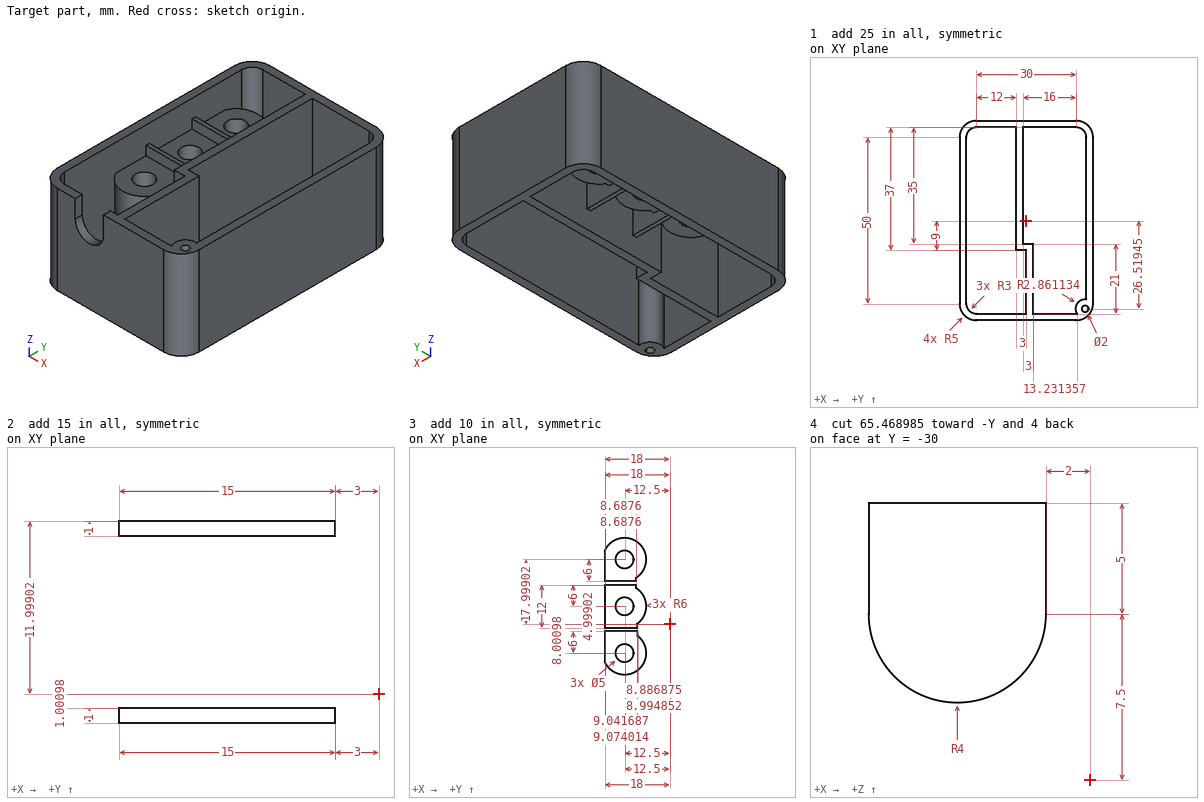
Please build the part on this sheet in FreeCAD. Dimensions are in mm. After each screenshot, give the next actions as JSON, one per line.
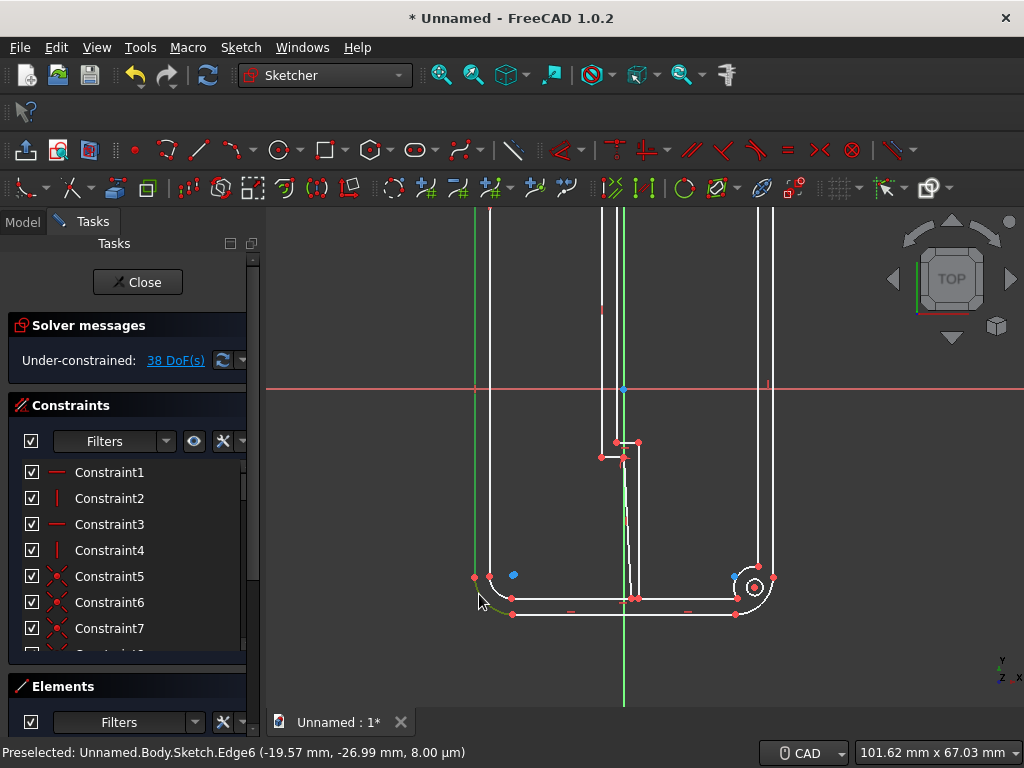
{"action": "left_click", "coordinate": [756, 150]}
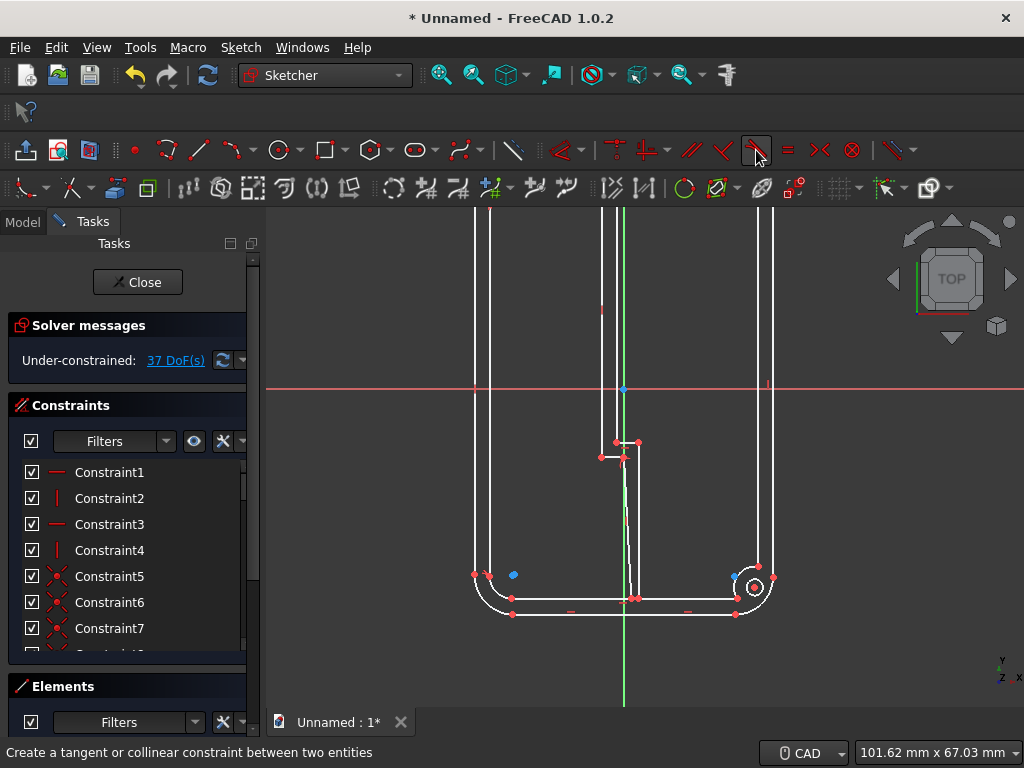
{"action": "left_click", "coordinate": [579, 615]}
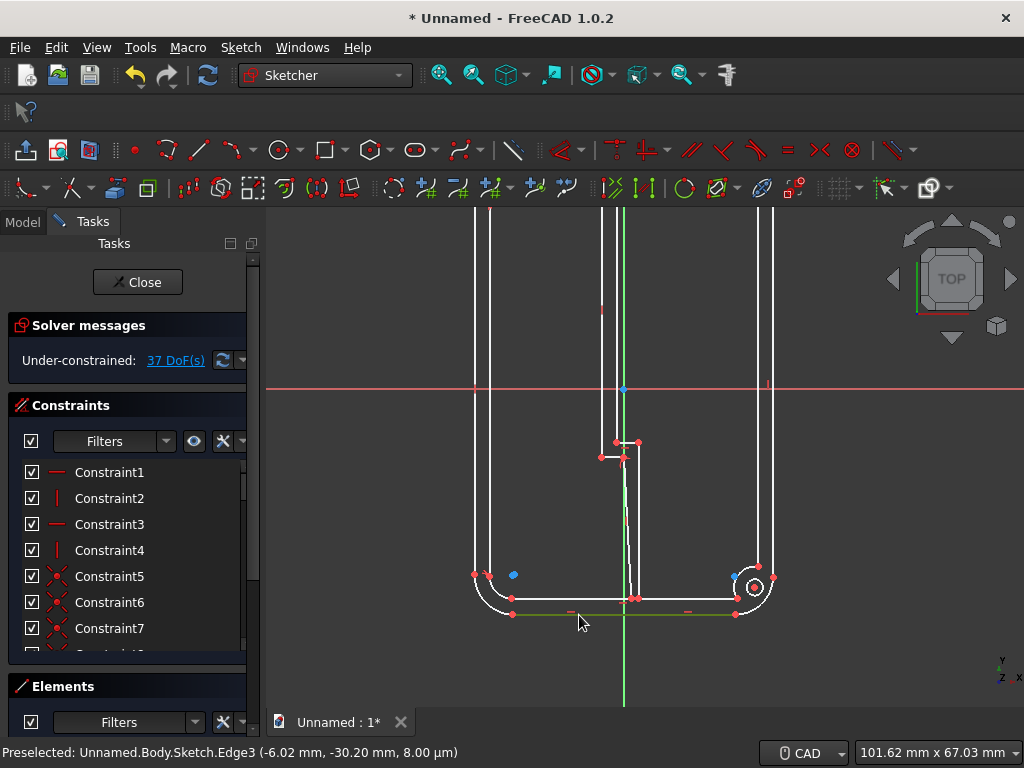
{"action": "left_click", "coordinate": [479, 592]}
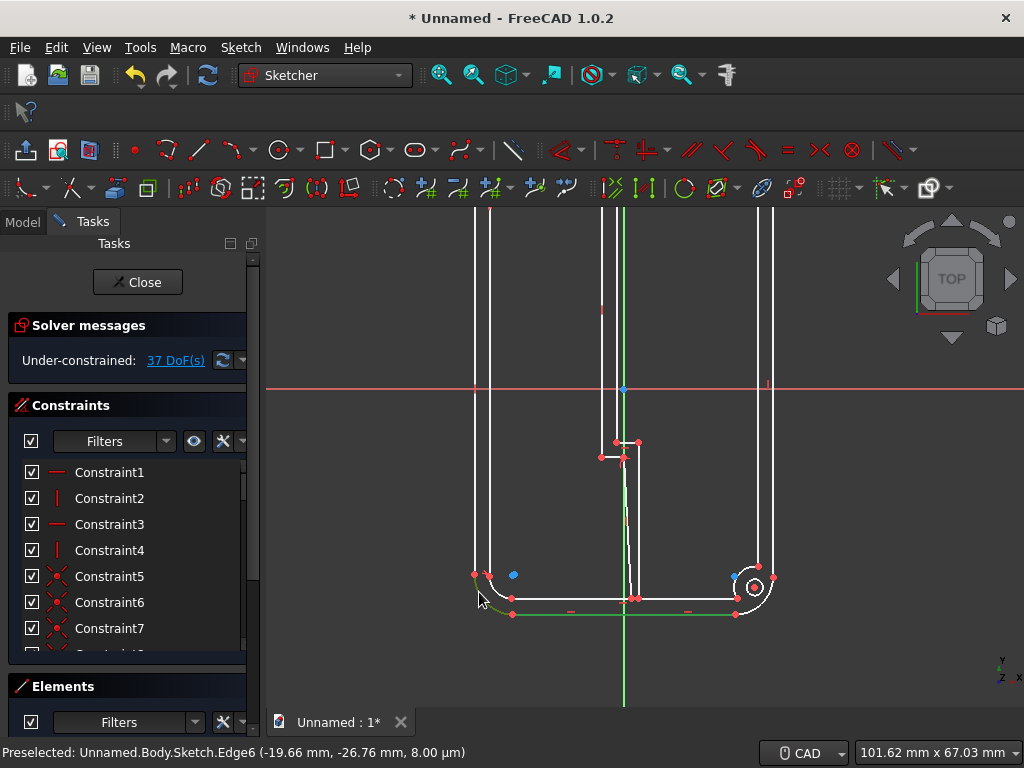
{"action": "left_click", "coordinate": [756, 150]}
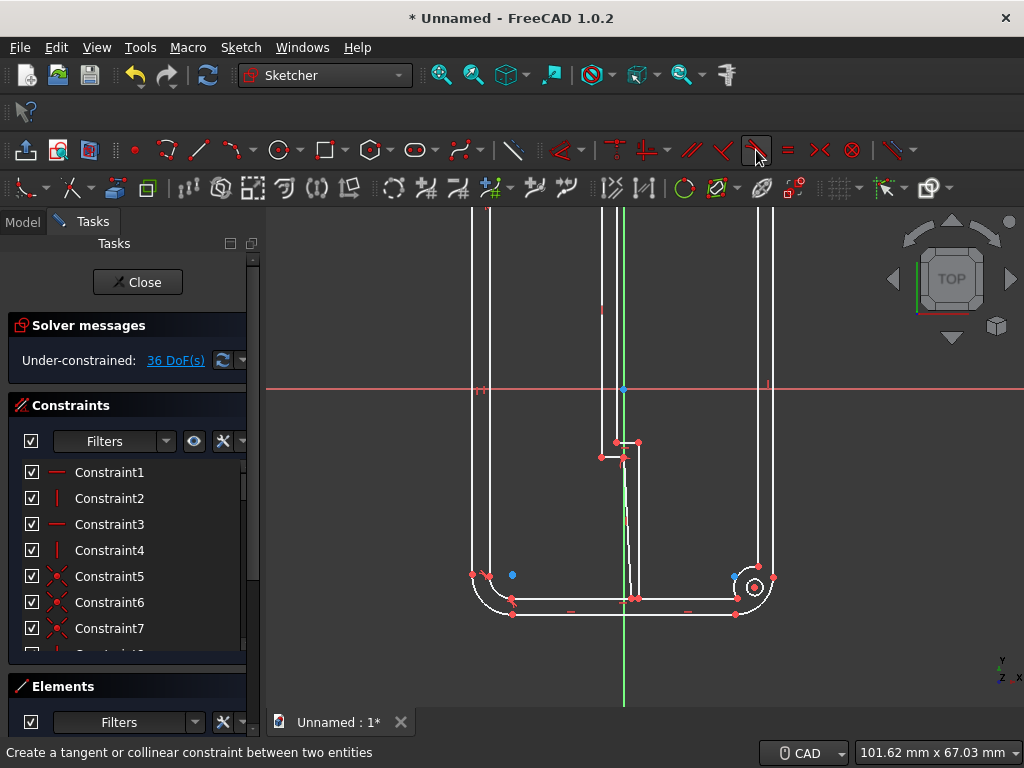
{"action": "left_click", "coordinate": [579, 615]}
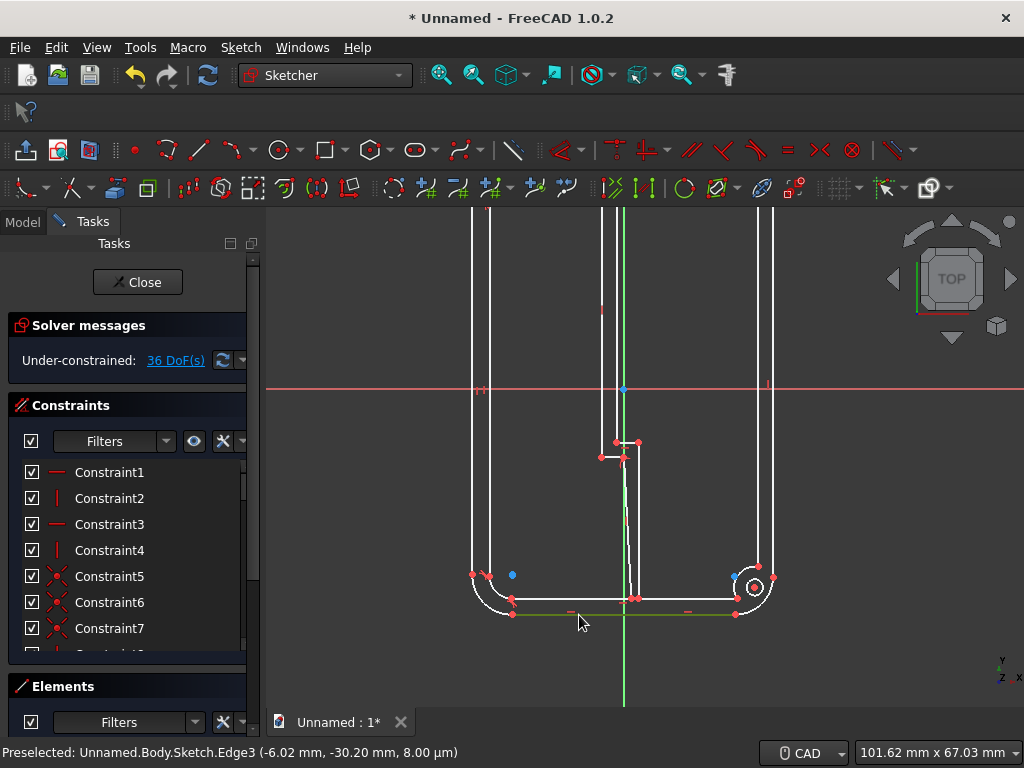
{"action": "left_click", "coordinate": [753, 610]}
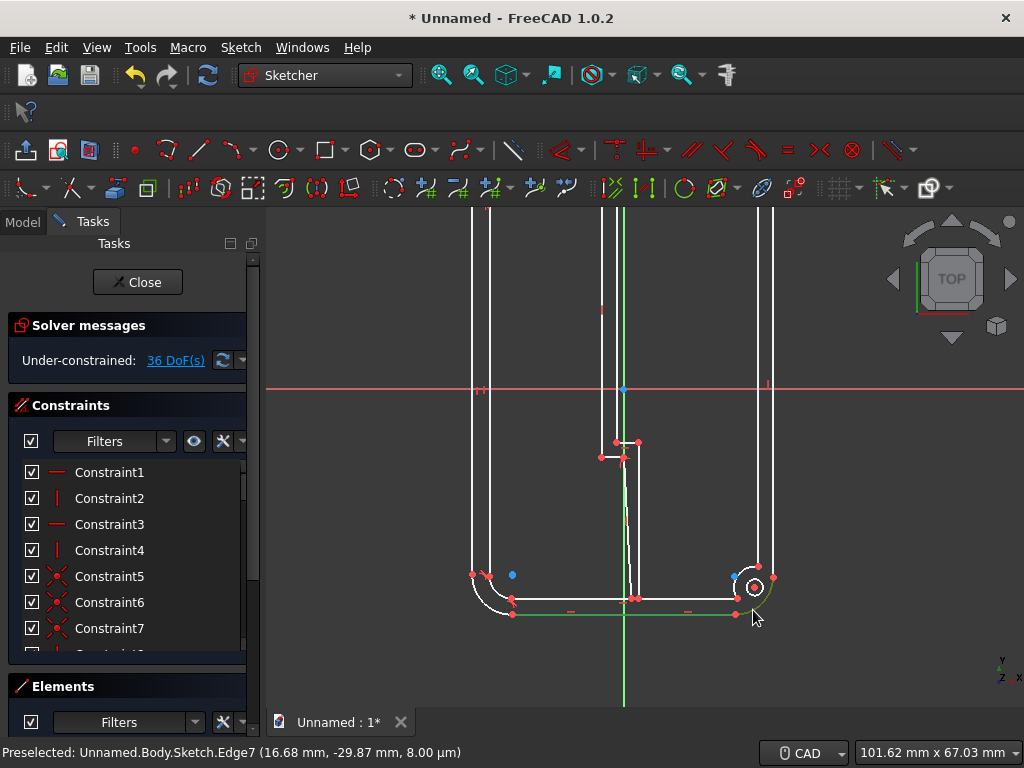
{"action": "left_click", "coordinate": [756, 150]}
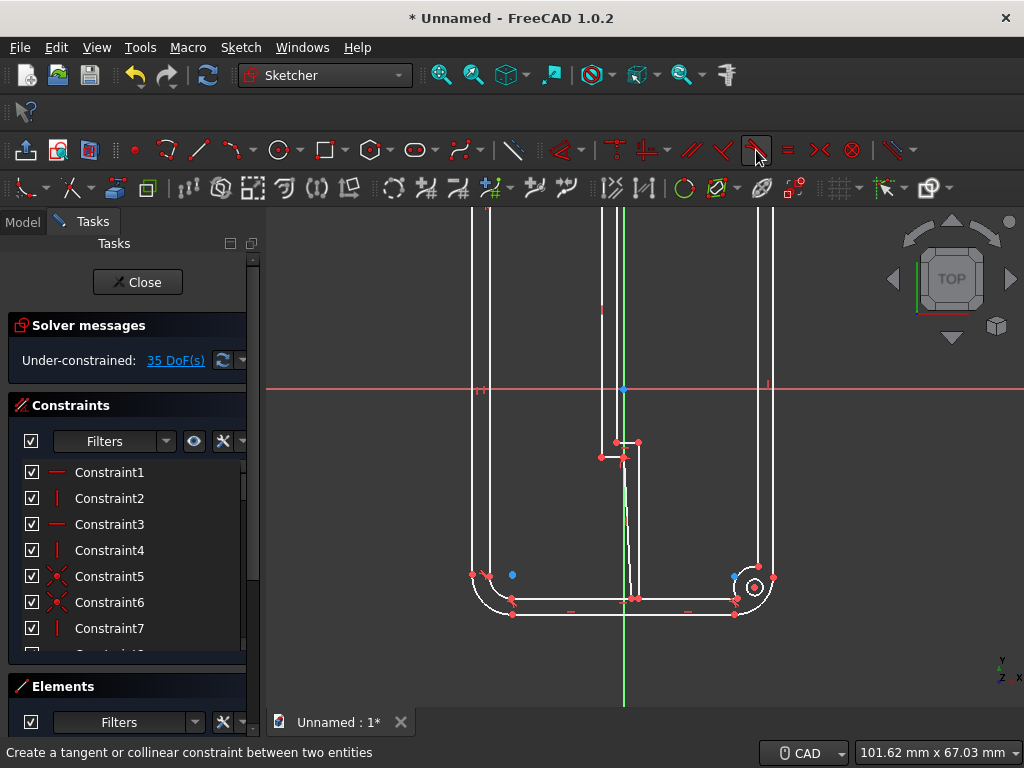
{"action": "left_click", "coordinate": [773, 466]}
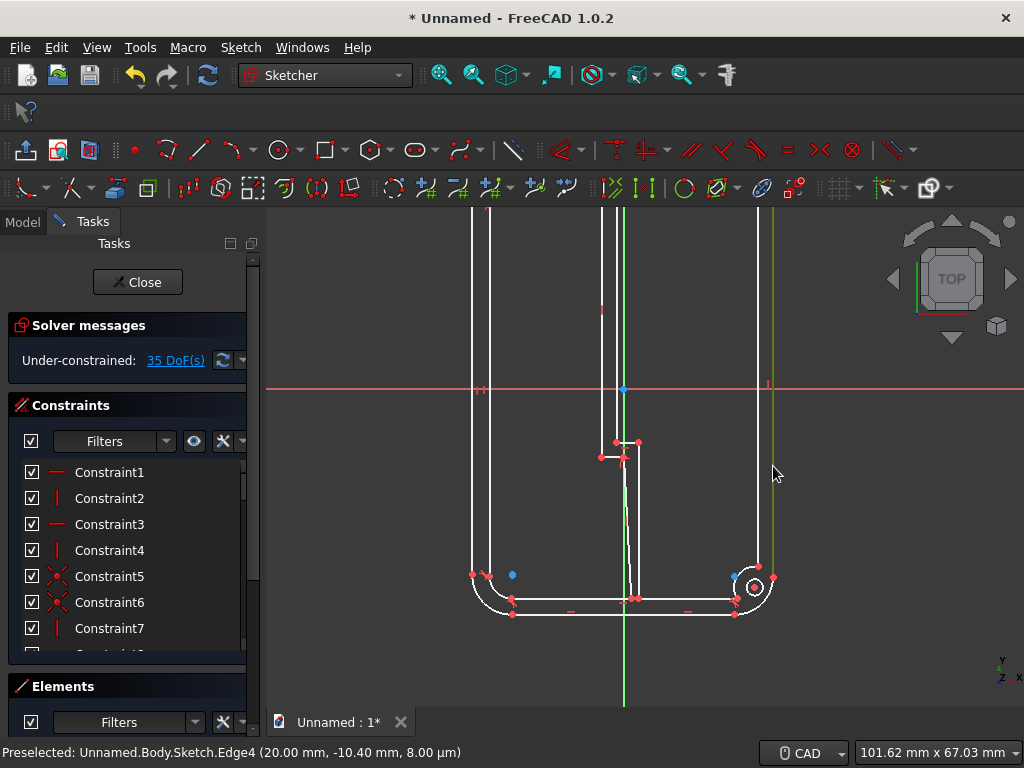
{"action": "left_click", "coordinate": [752, 611]}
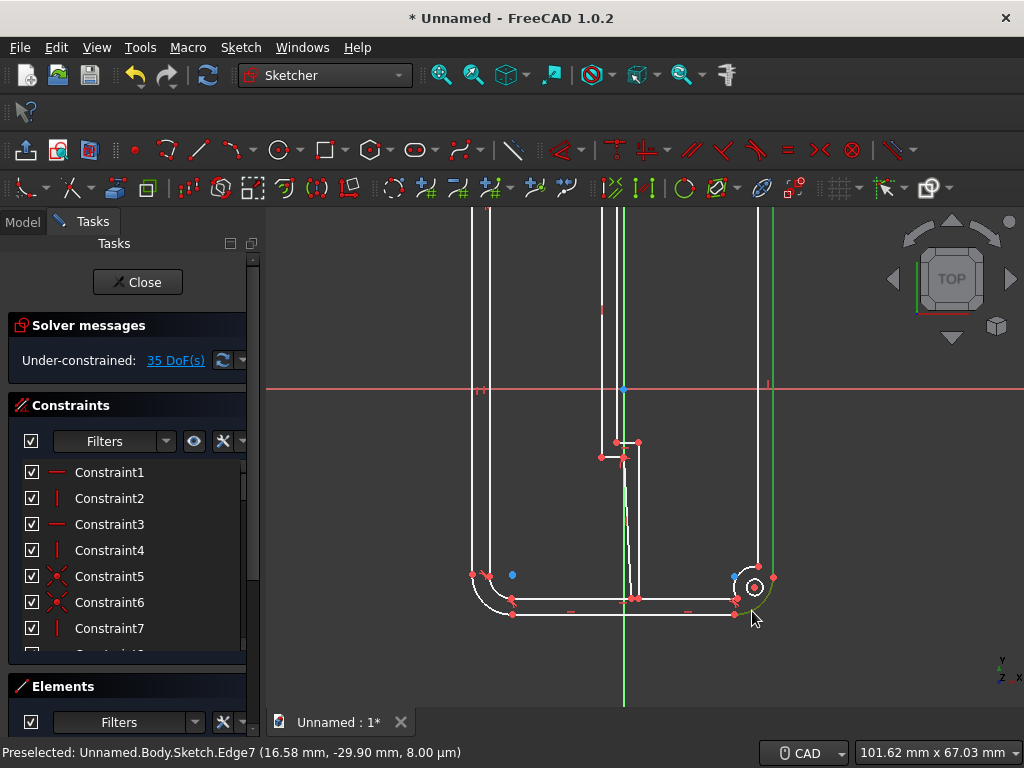
{"action": "left_click", "coordinate": [756, 150]}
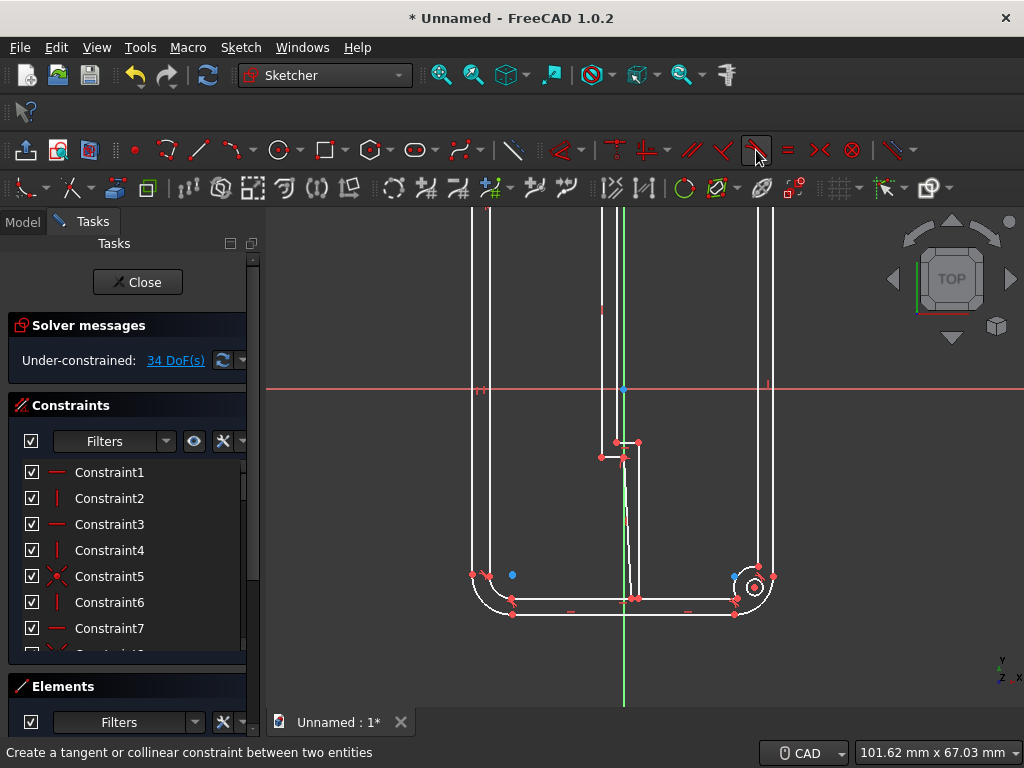
{"action": "left_click", "coordinate": [773, 465]}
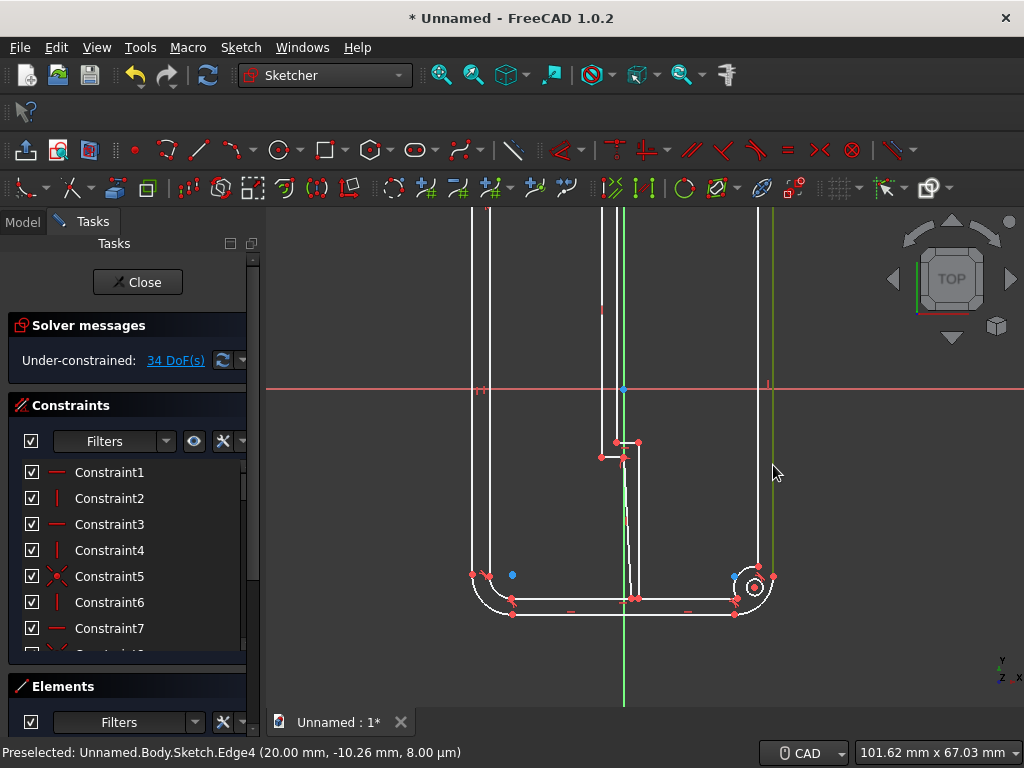
{"action": "scroll", "coordinate": [480, 594], "scroll_direction": "down", "scroll_amount": 2}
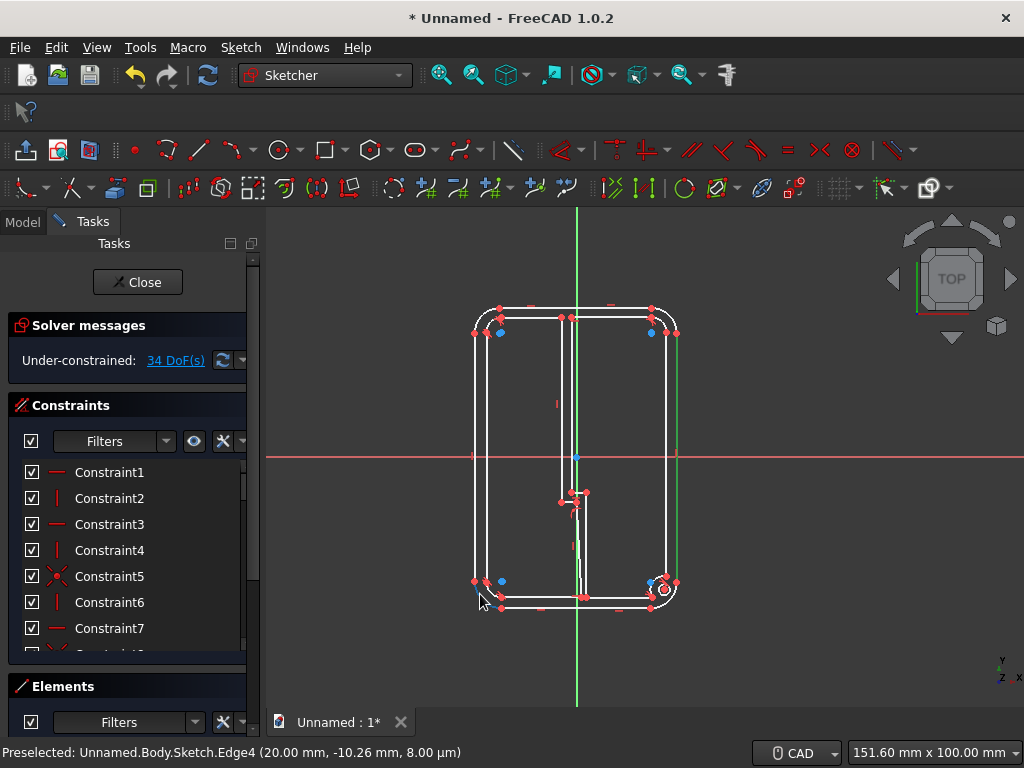
{"action": "scroll", "coordinate": [674, 322], "scroll_direction": "up", "scroll_amount": 2}